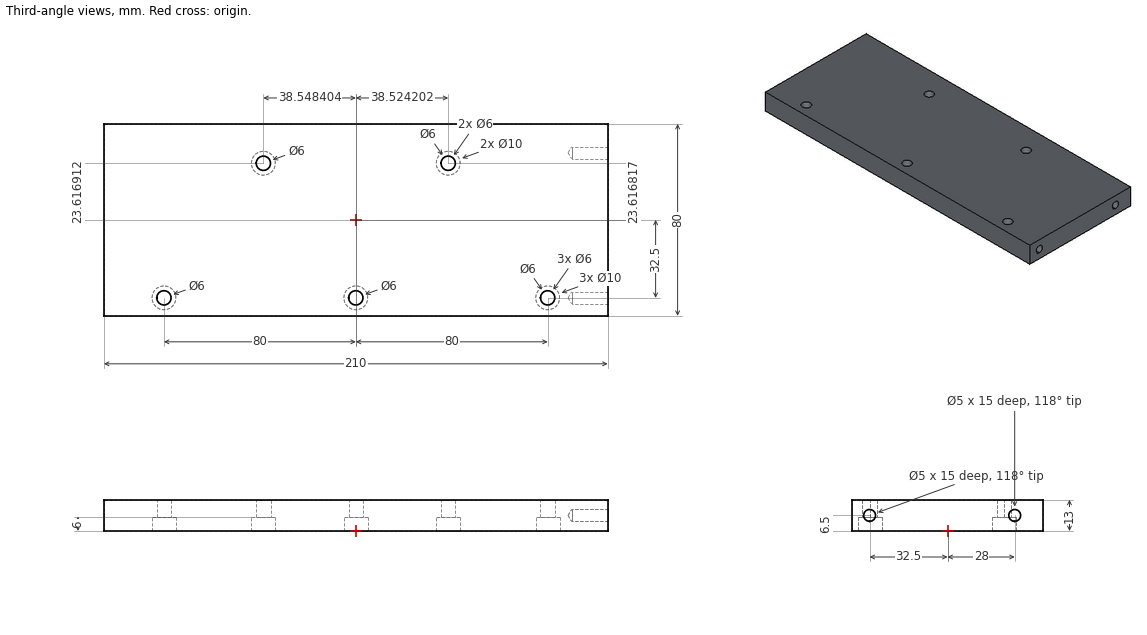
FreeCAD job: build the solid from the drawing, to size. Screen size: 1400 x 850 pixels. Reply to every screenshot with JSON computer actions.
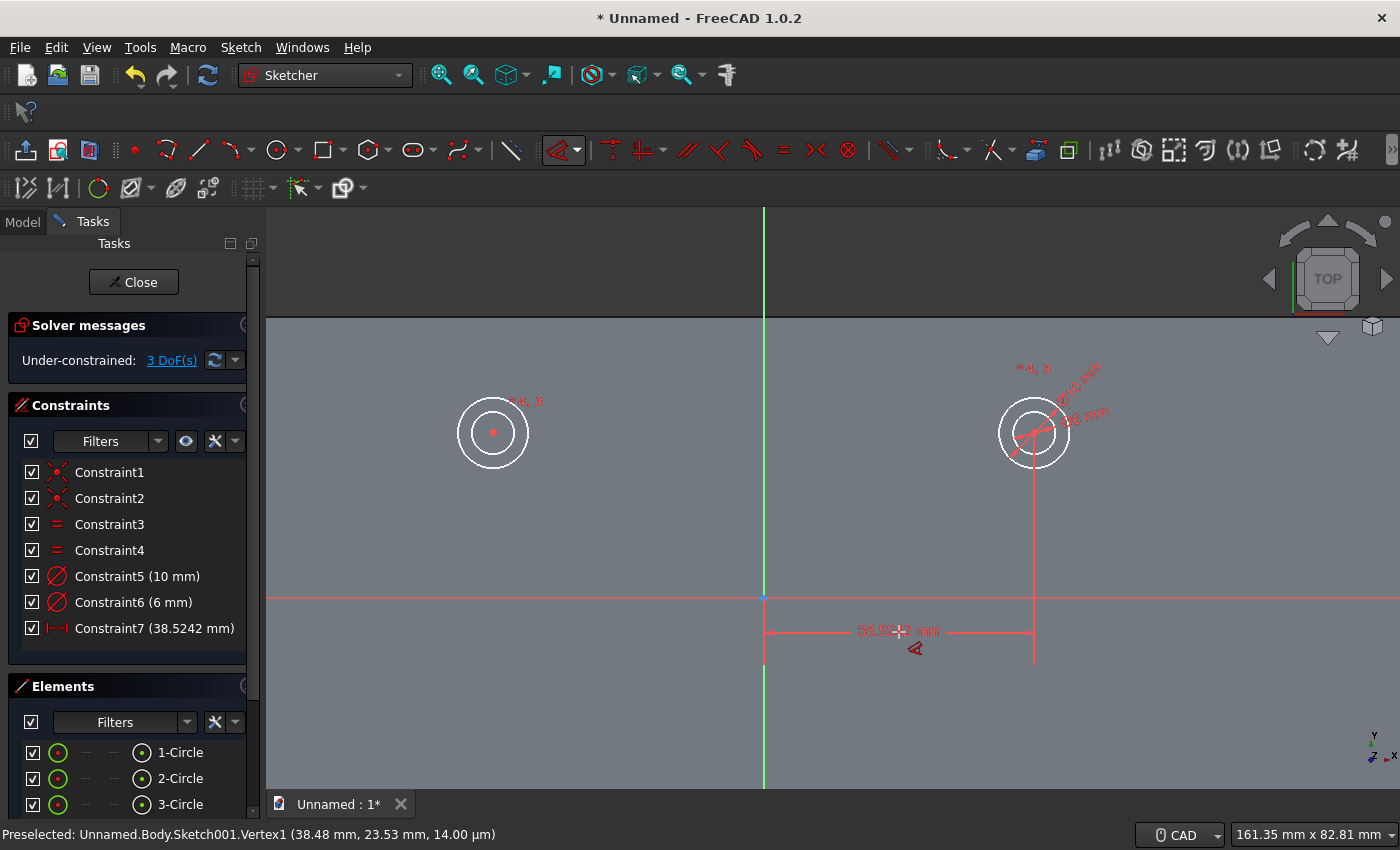
{"action": "left_click", "coordinate": [1034, 433]}
{"action": "left_click", "coordinate": [1068, 516]}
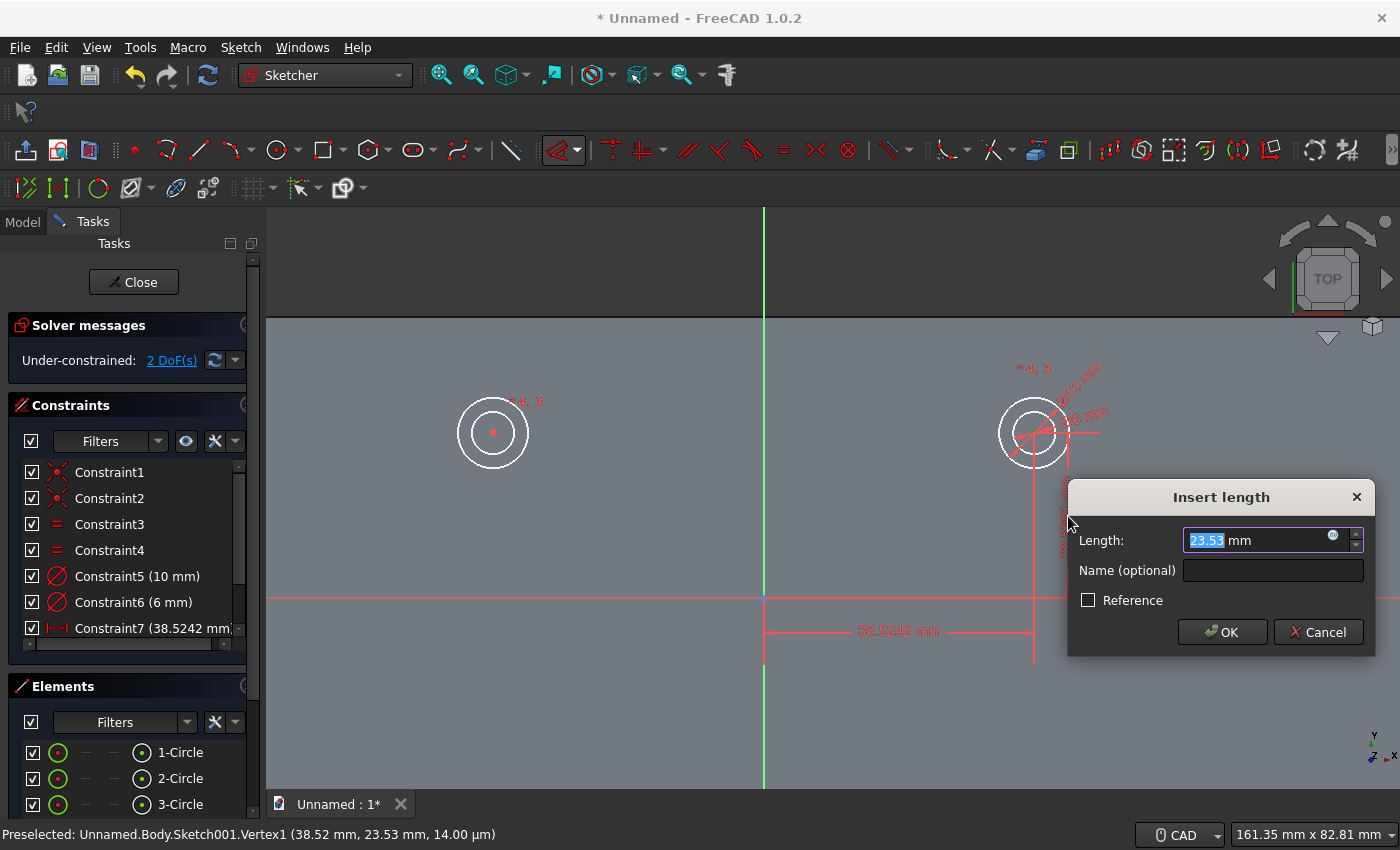
{"action": "type", "text": "23.616817"}
{"action": "key", "text": "Return"}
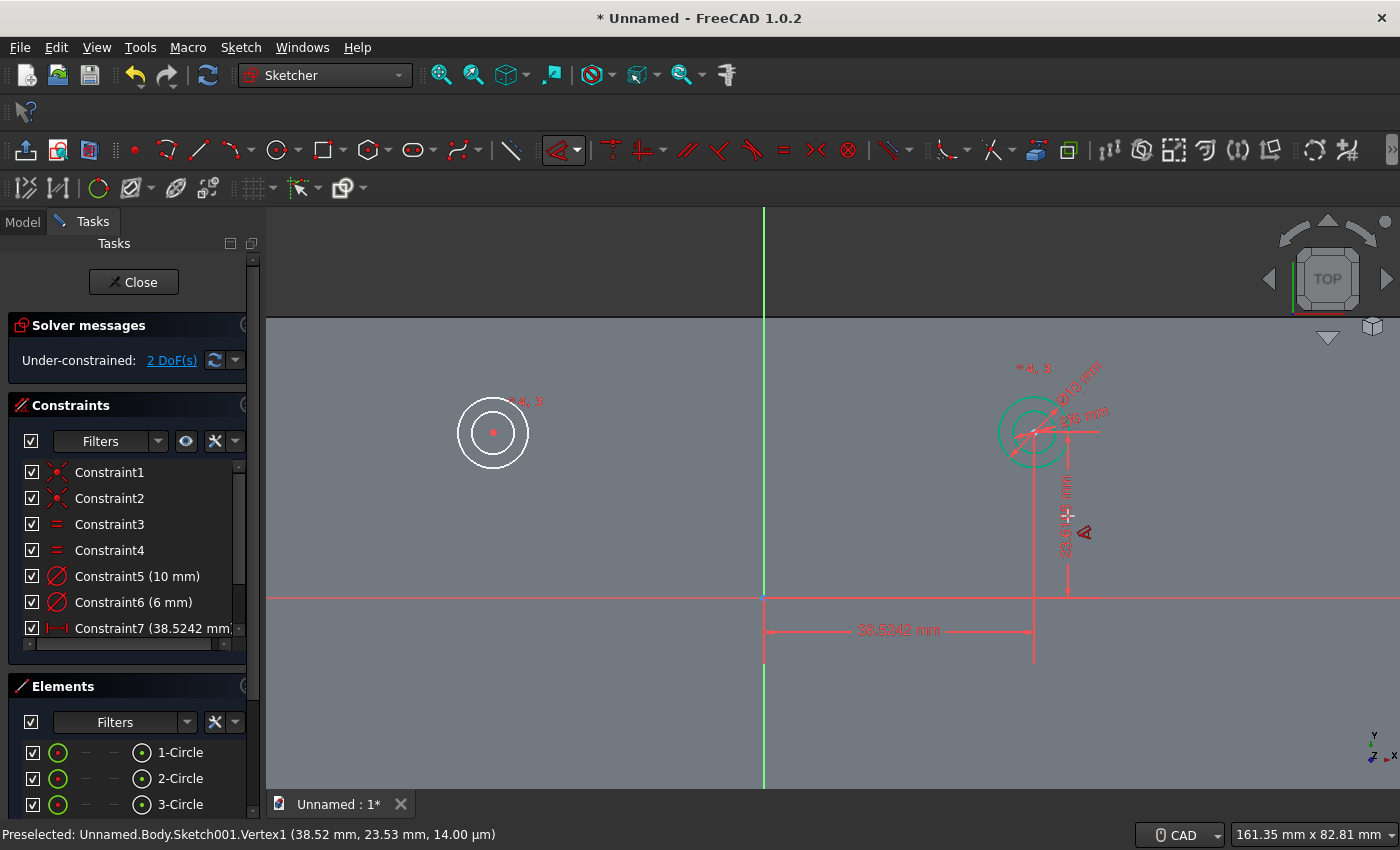
{"action": "left_click", "coordinate": [493, 433]}
{"action": "left_click", "coordinate": [628, 632]}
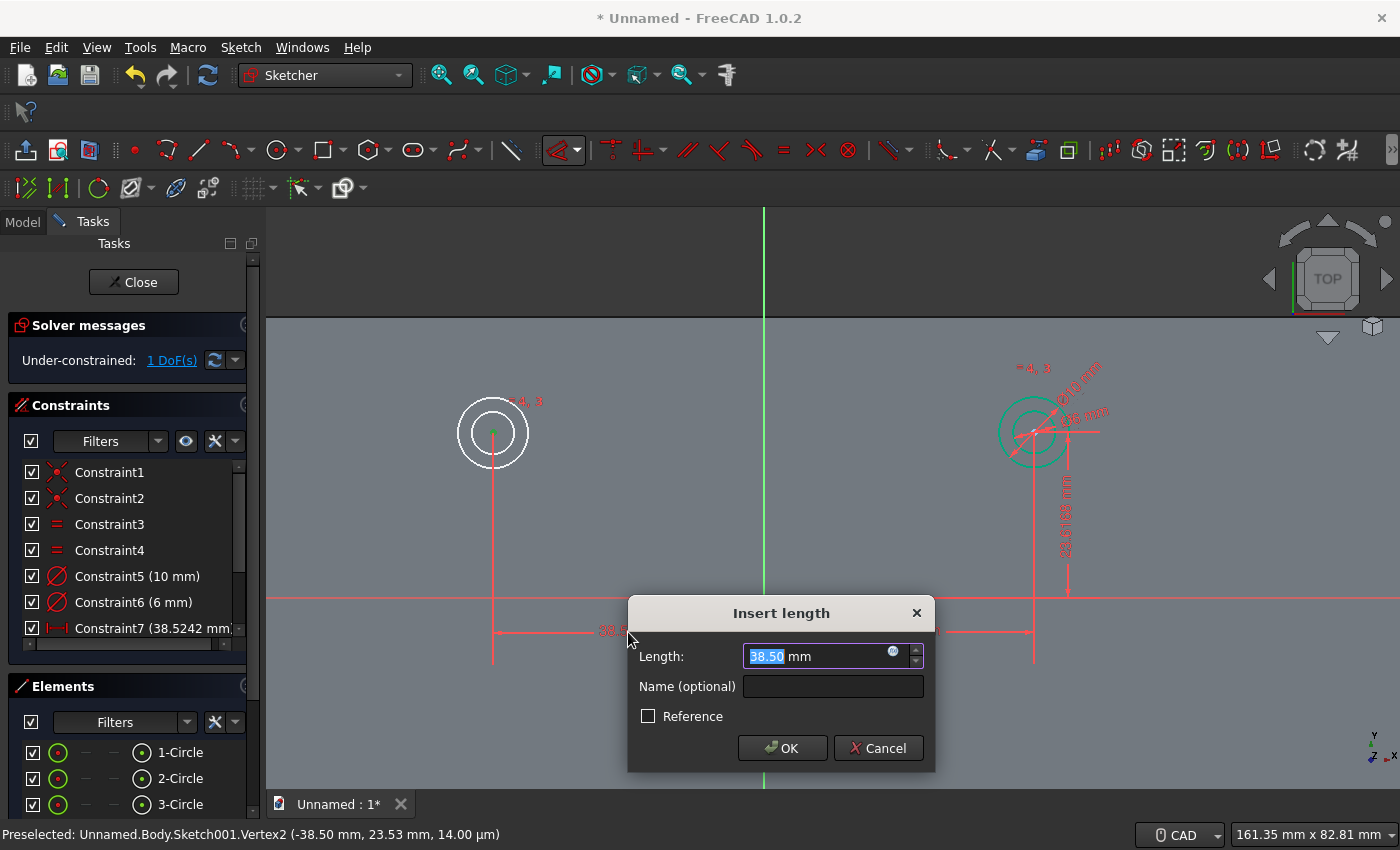
{"action": "type", "text": "38.548404"}
{"action": "key", "text": "Return"}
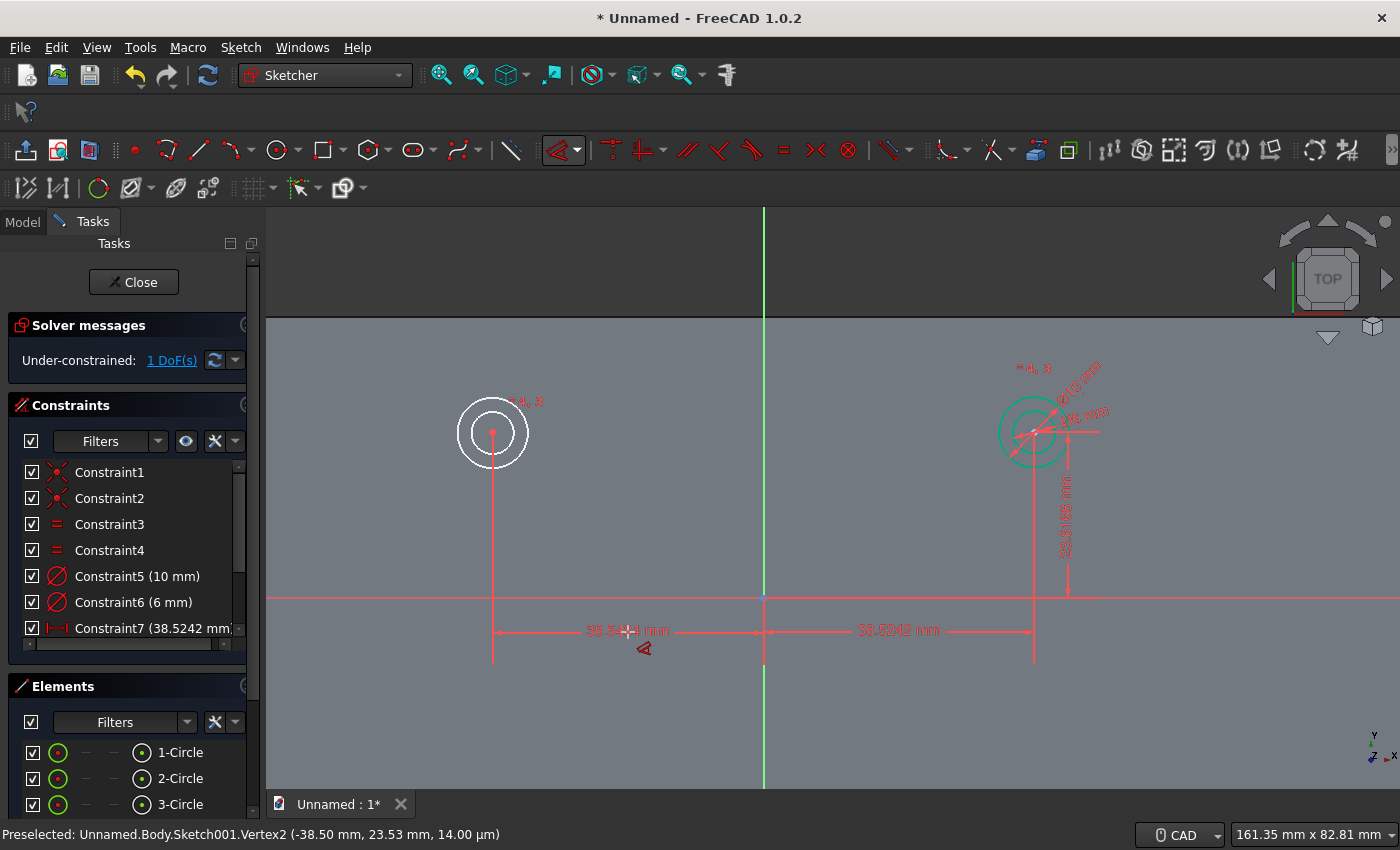
{"action": "left_click", "coordinate": [493, 433]}
{"action": "left_click", "coordinate": [459, 516]}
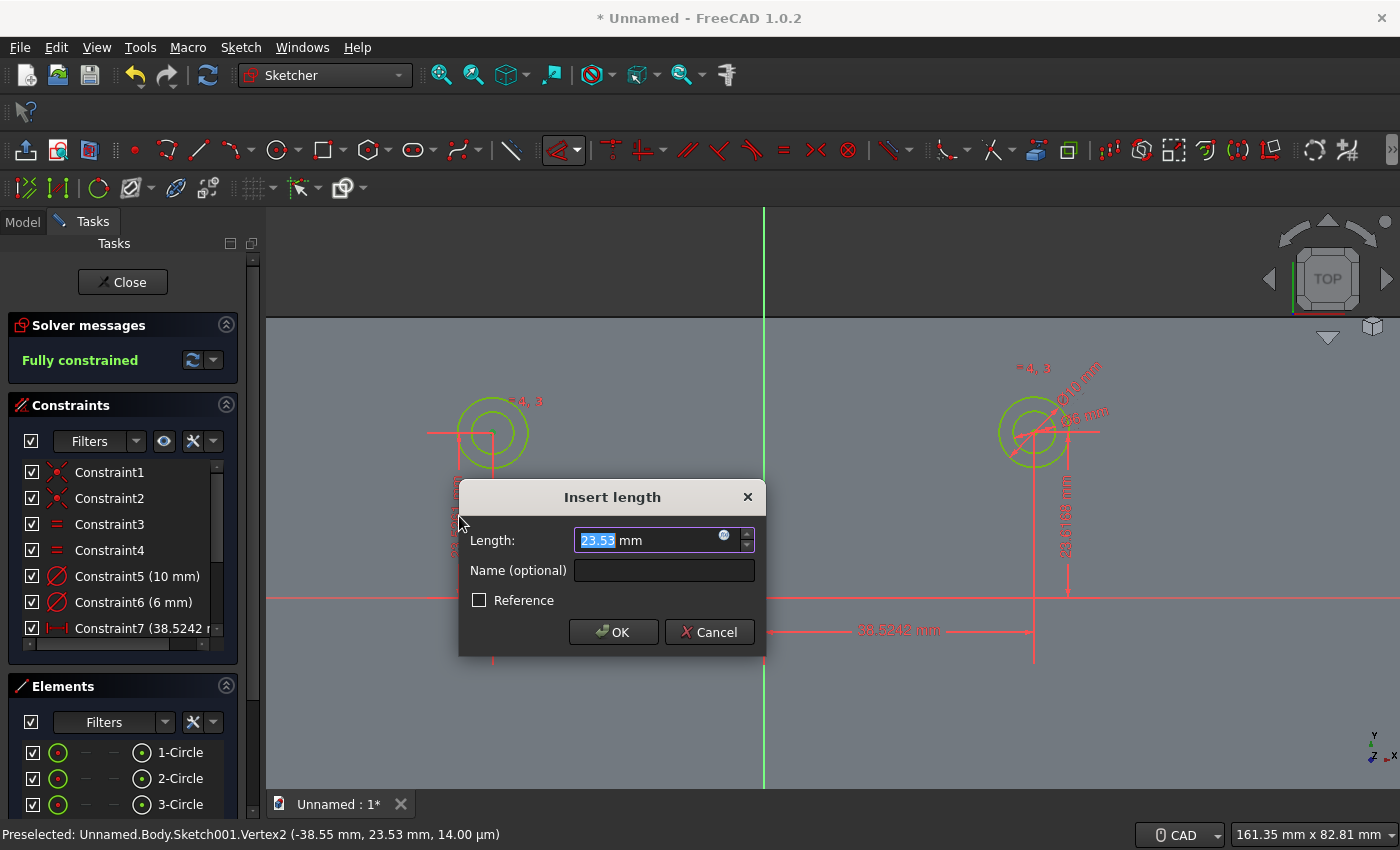
{"action": "type", "text": "23.616912"}
{"action": "key", "text": "Return"}
{"action": "key", "text": "Escape"}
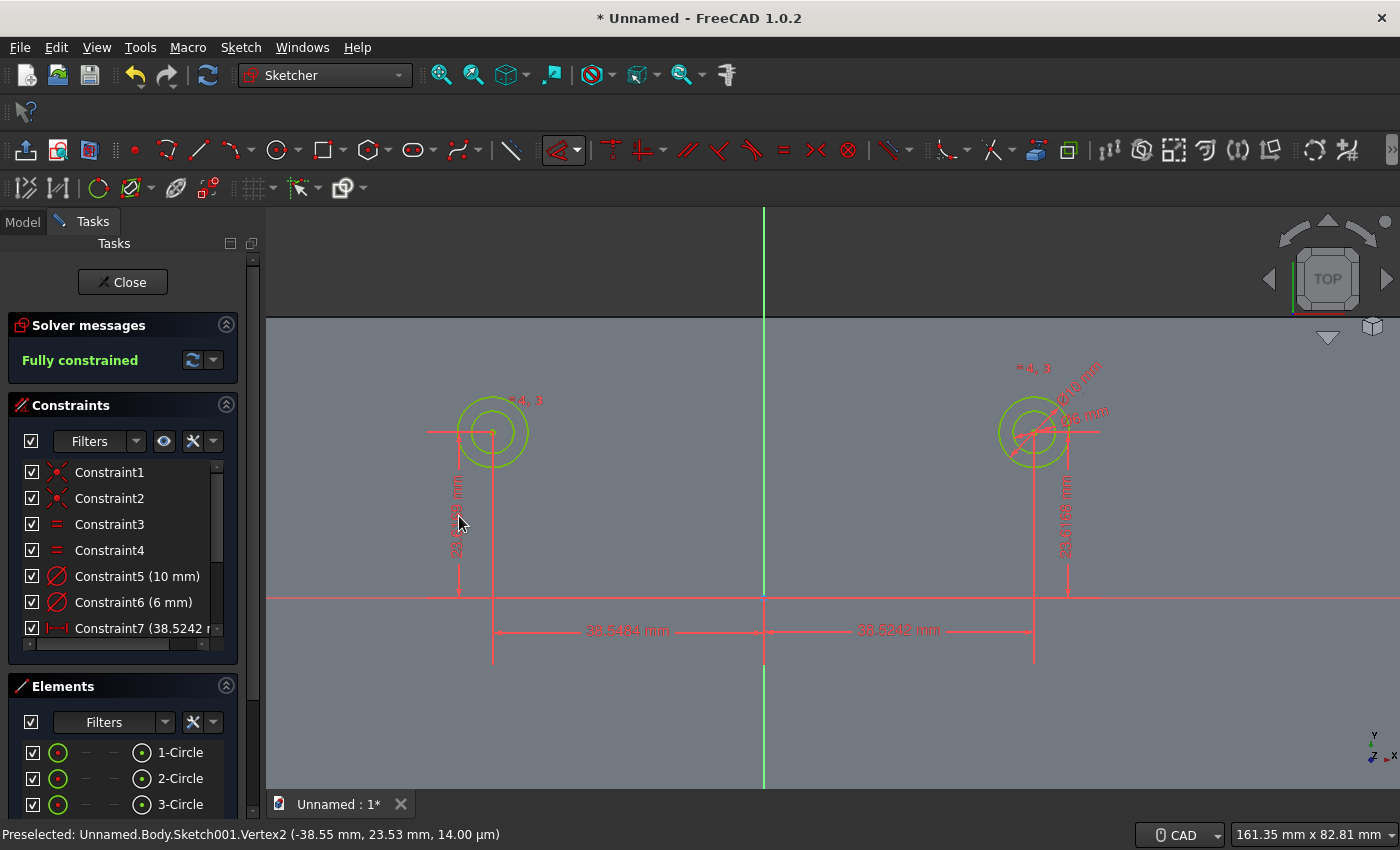
{"action": "left_click", "coordinate": [123, 282]}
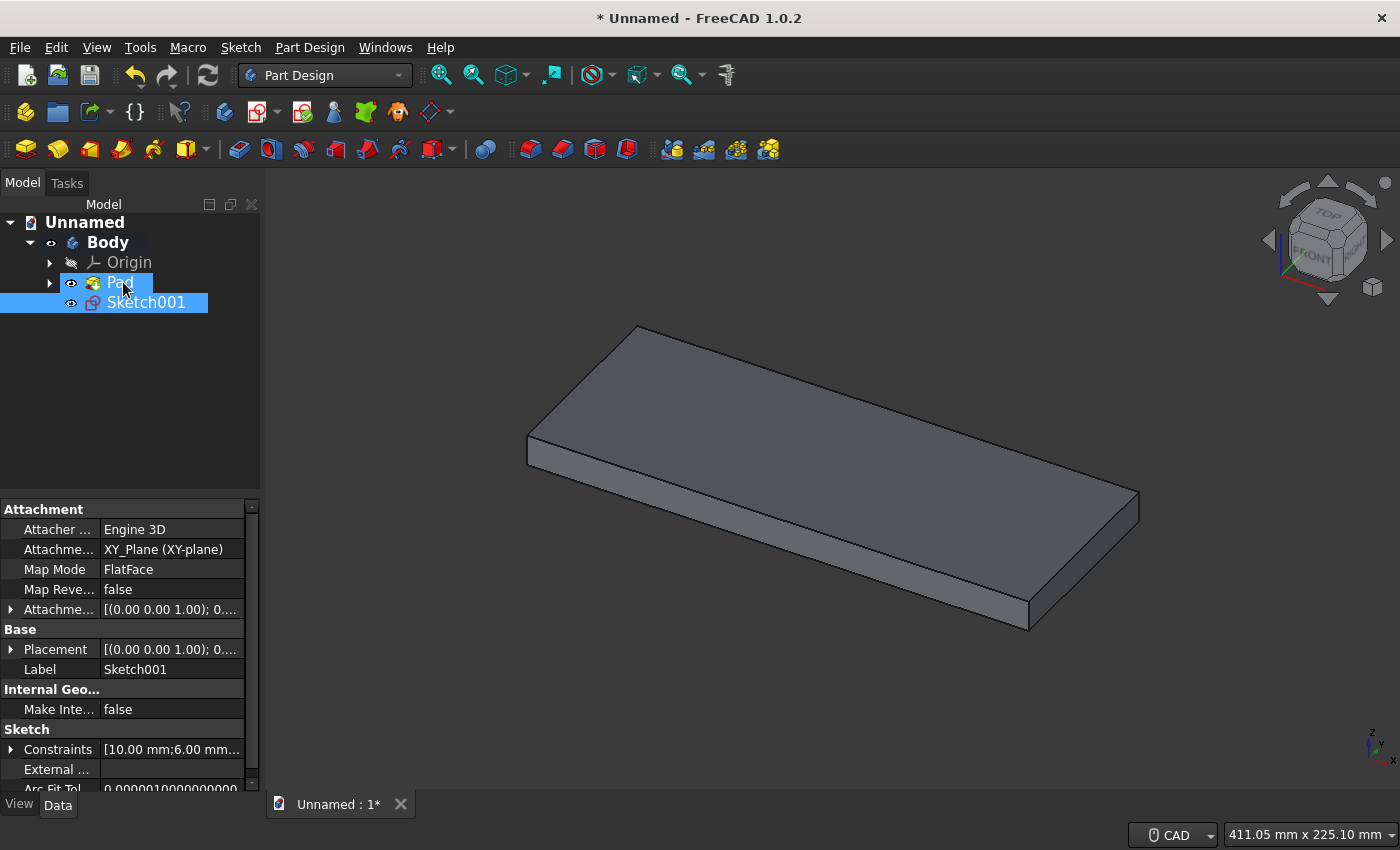
{"action": "left_click", "coordinate": [240, 150]}